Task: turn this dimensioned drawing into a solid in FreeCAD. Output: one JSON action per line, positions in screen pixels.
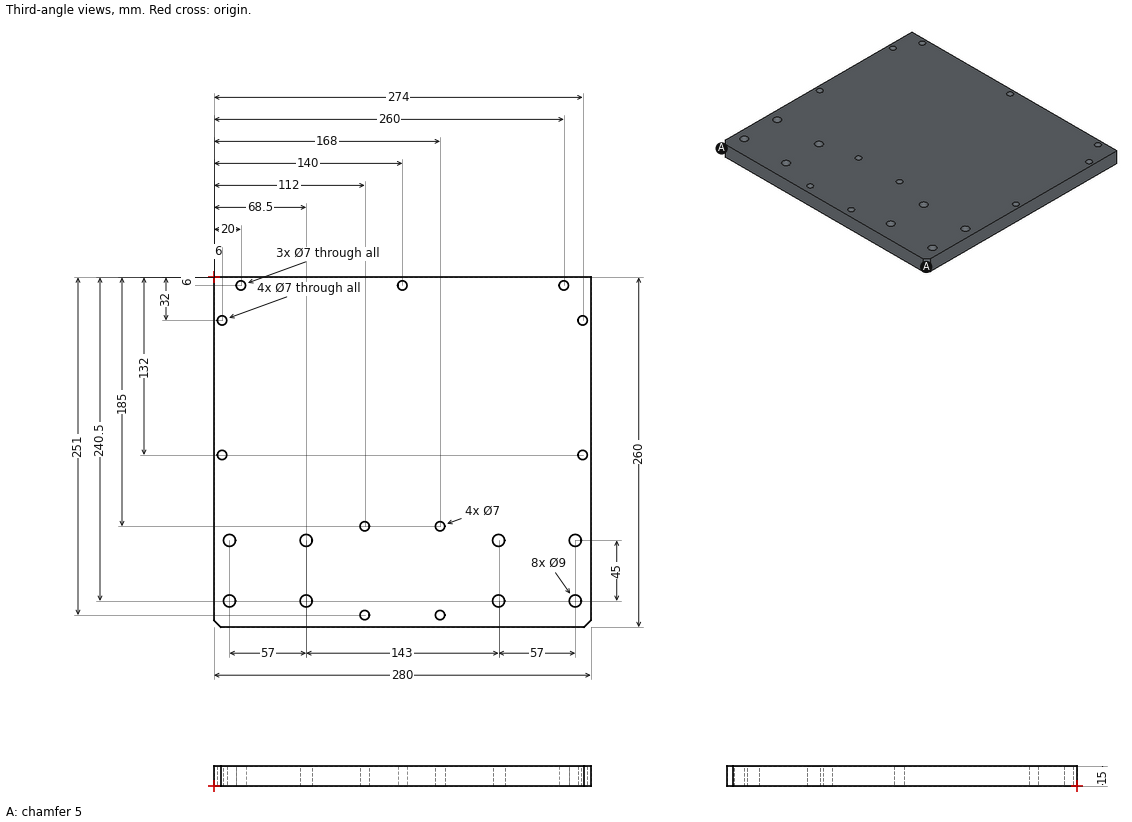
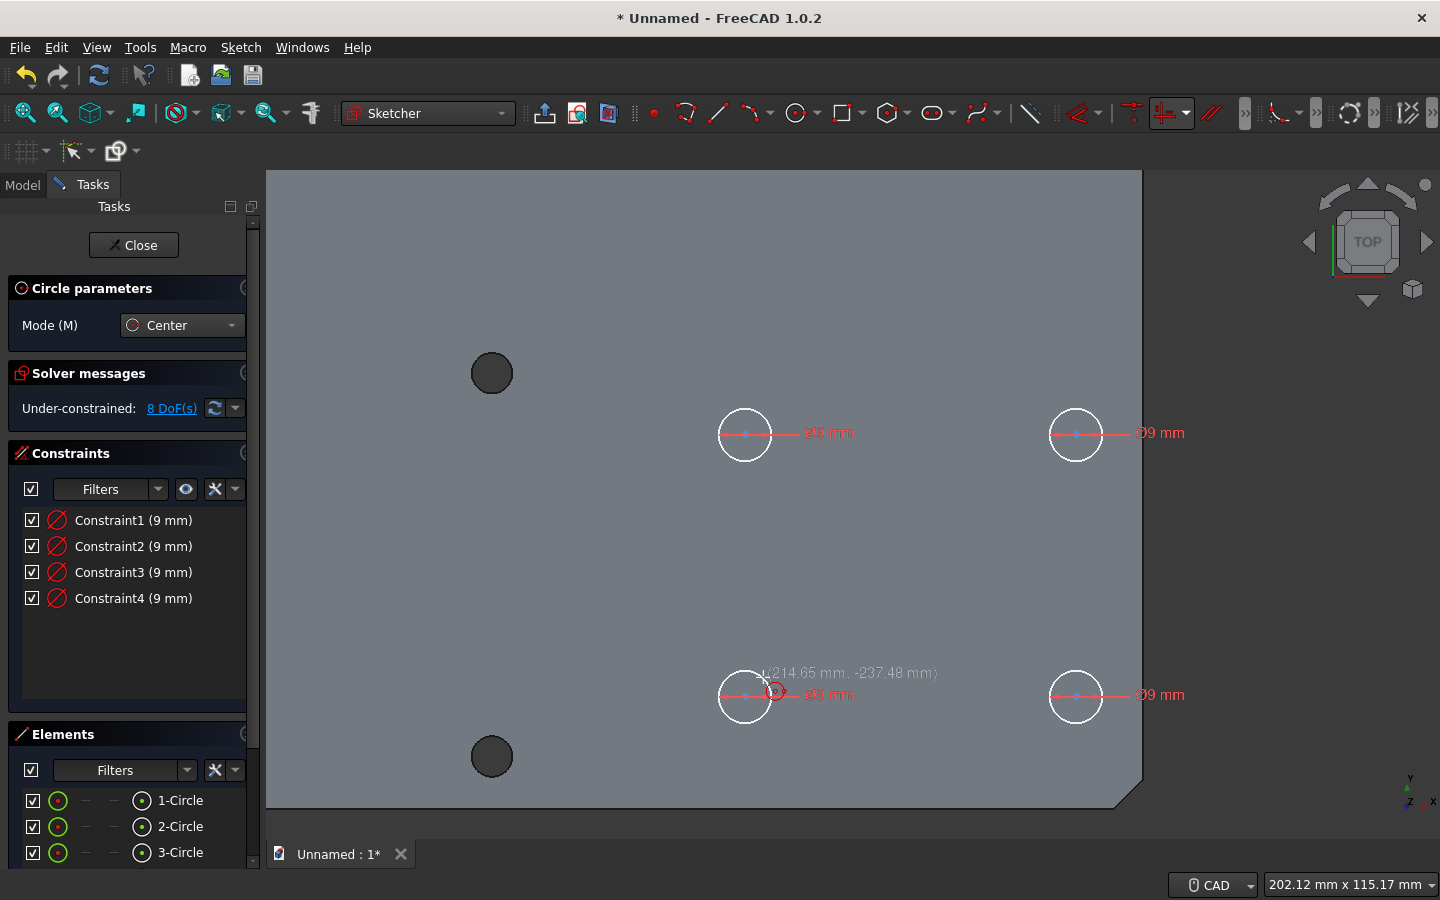
{"action": "scroll", "coordinate": [989, 718], "scroll_direction": "down", "scroll_amount": 6}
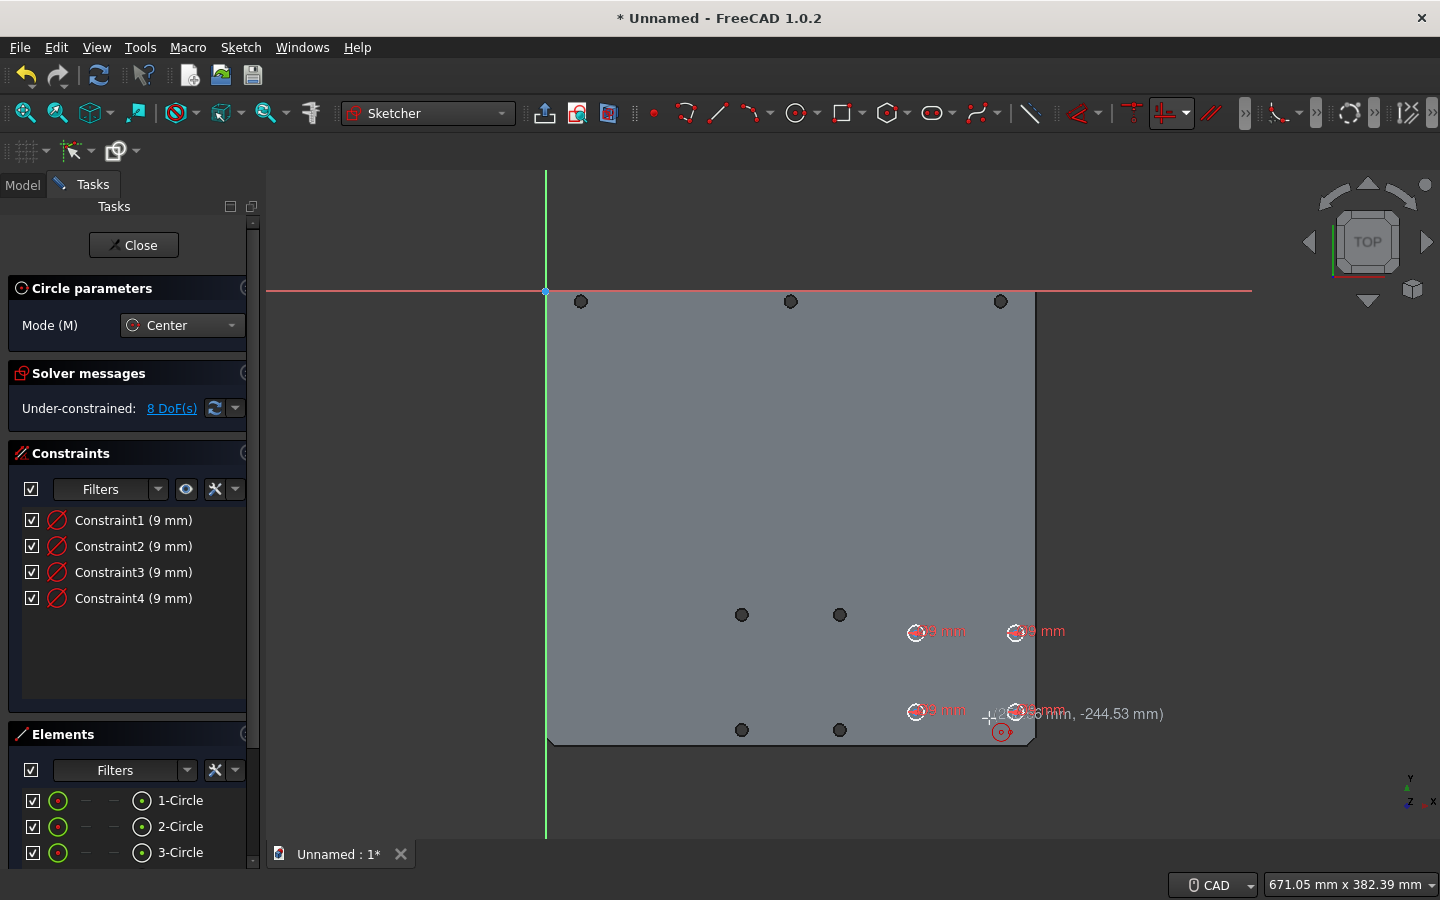
{"action": "scroll", "coordinate": [666, 712], "scroll_direction": "up", "scroll_amount": 6}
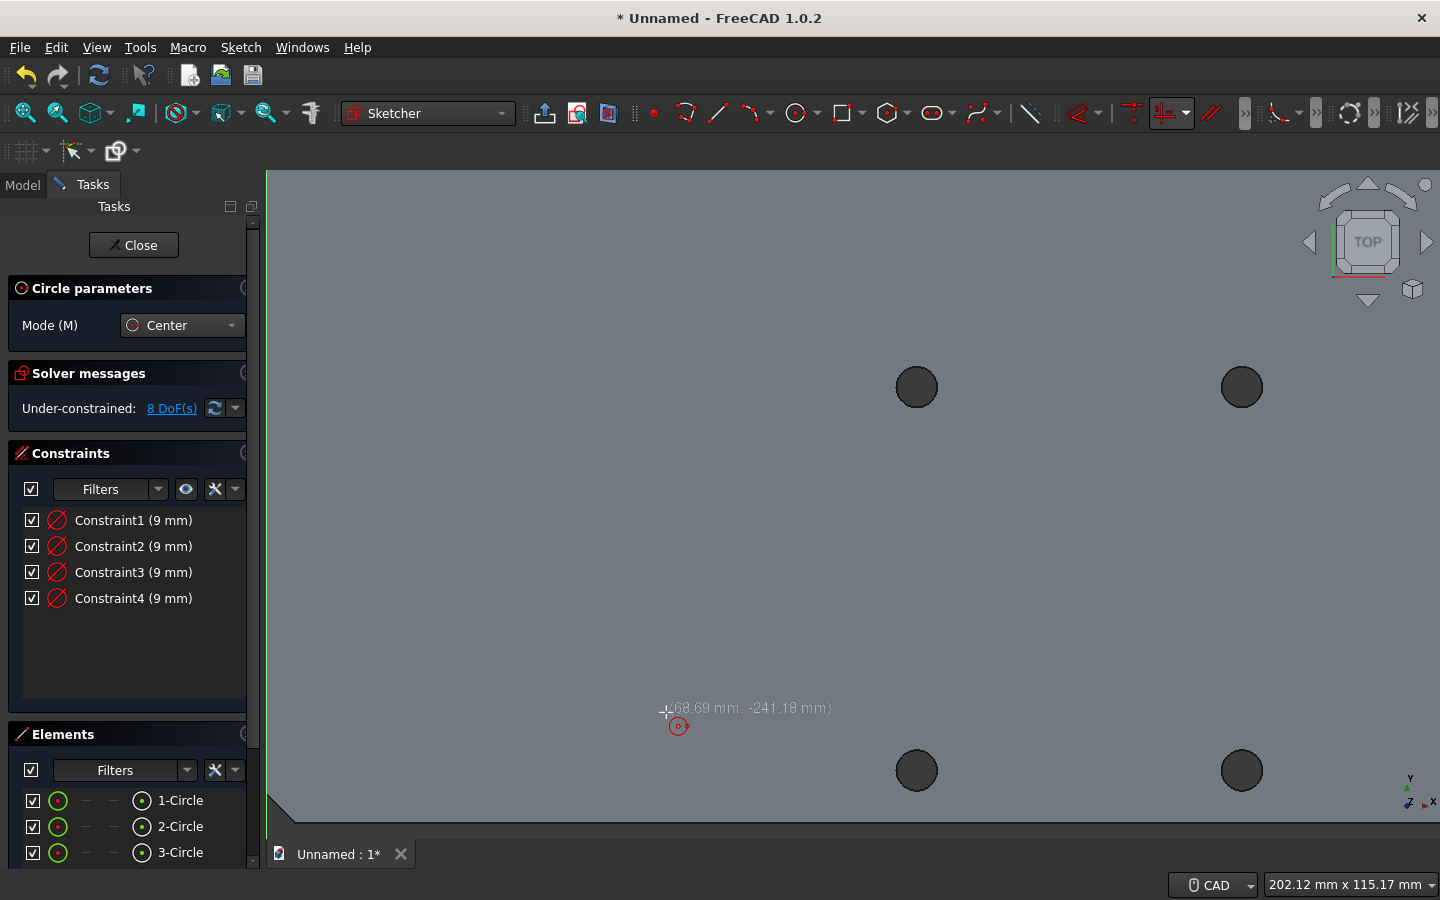
{"action": "left_click", "coordinate": [664, 710]}
{"action": "mouse_move", "coordinate": [683, 691]}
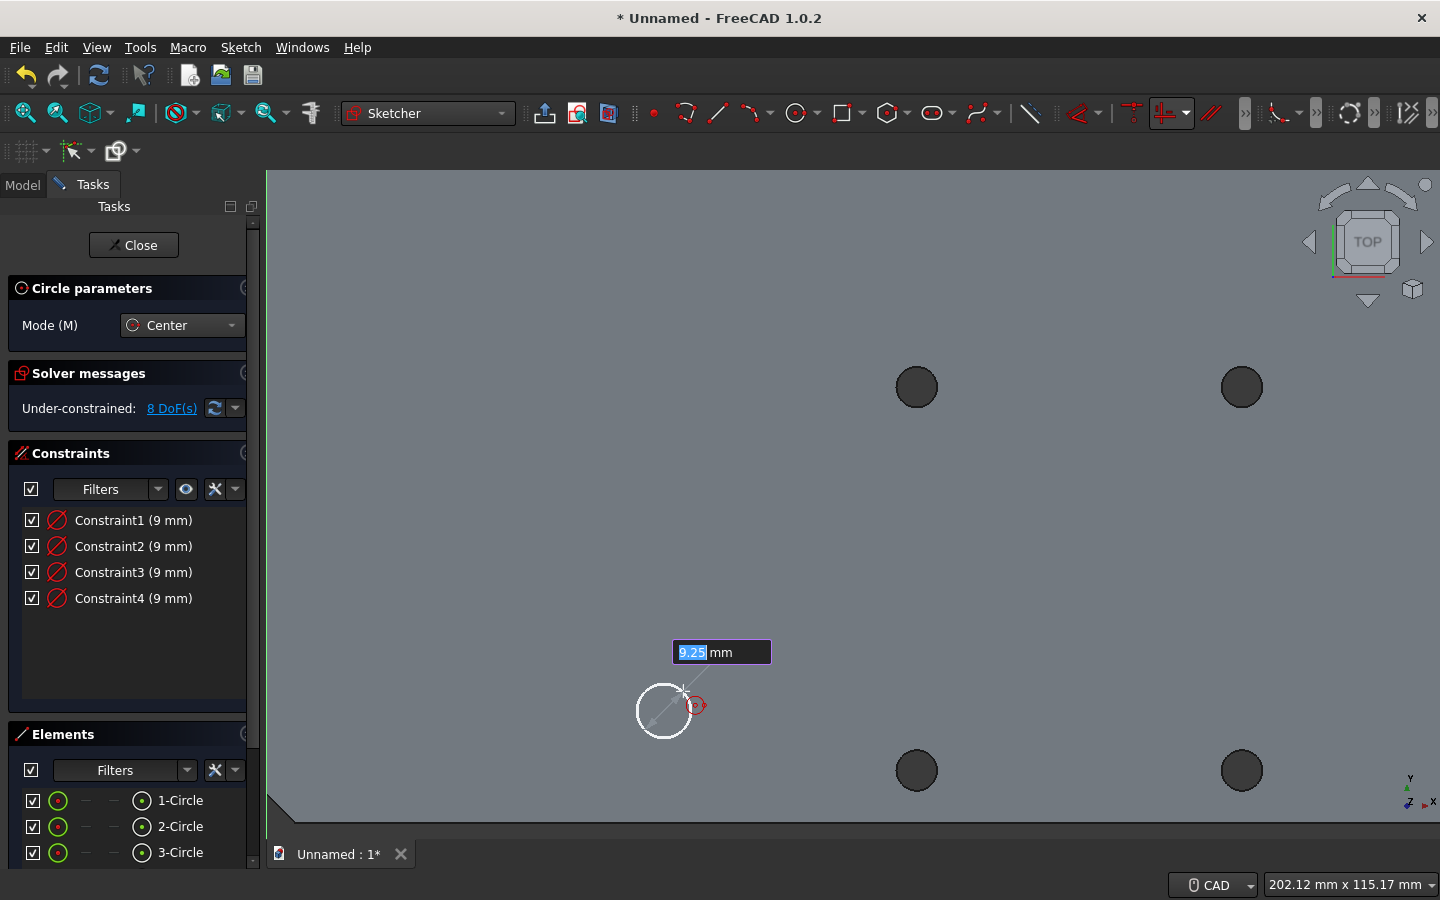
{"action": "type", "text": "9"}
{"action": "key", "text": "Return"}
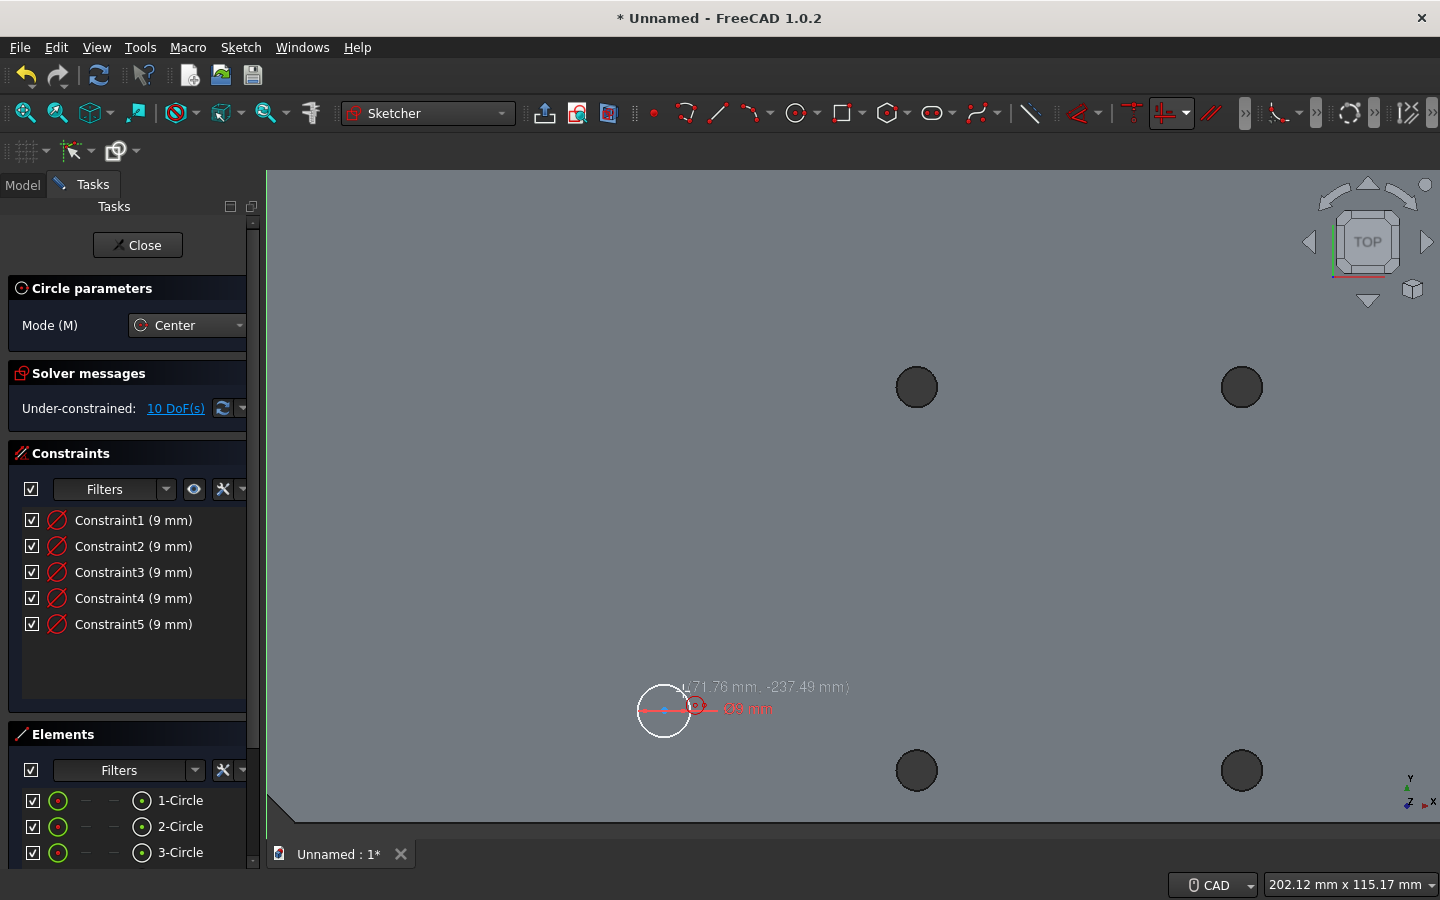
{"action": "left_click", "coordinate": [664, 448]}
{"action": "mouse_move", "coordinate": [683, 430]}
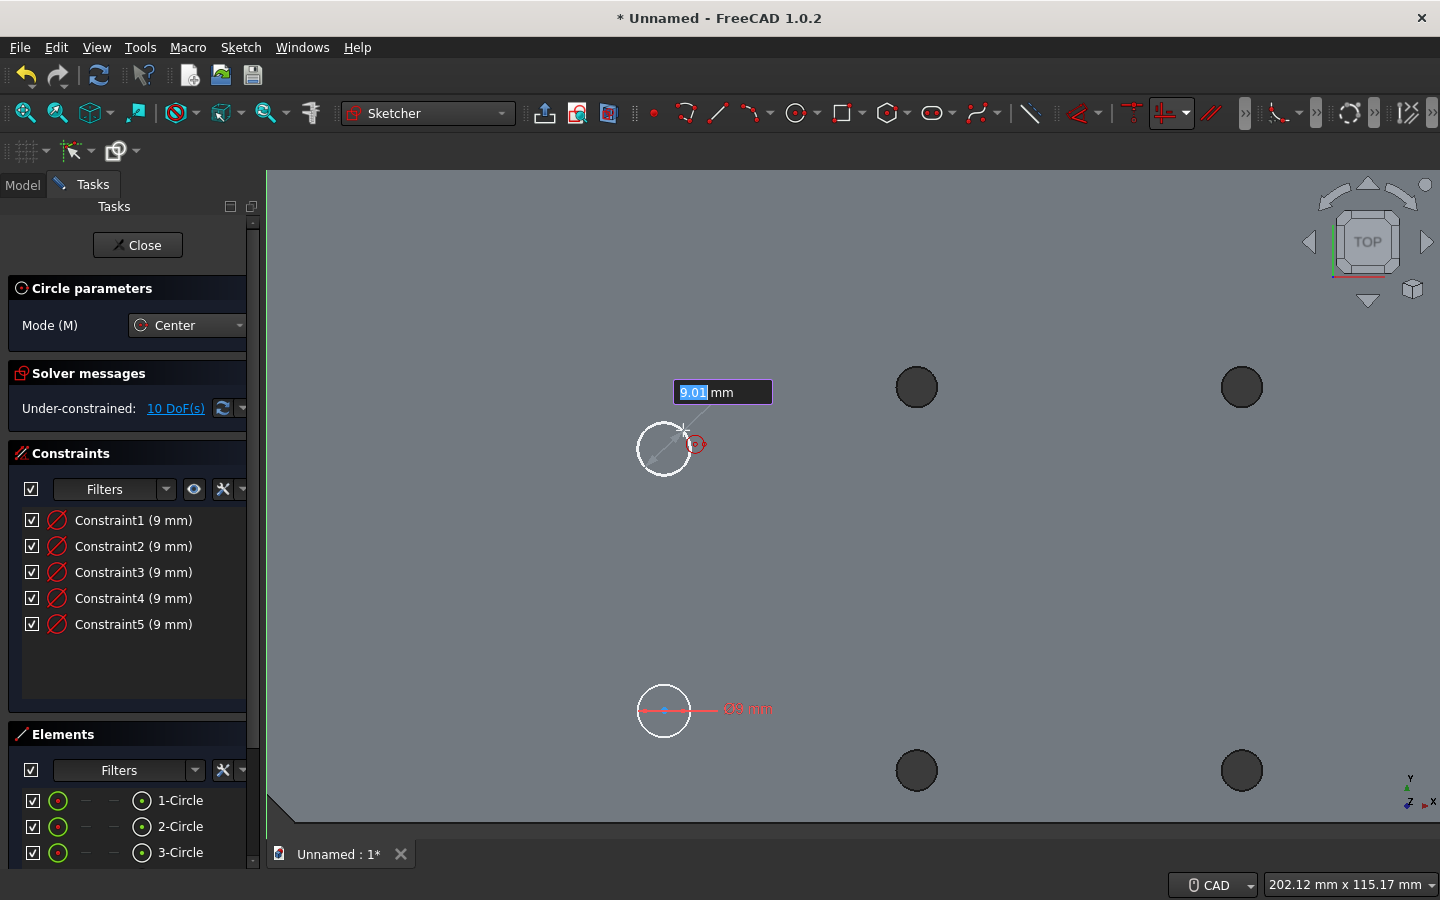
{"action": "type", "text": "9"}
{"action": "key", "text": "Return"}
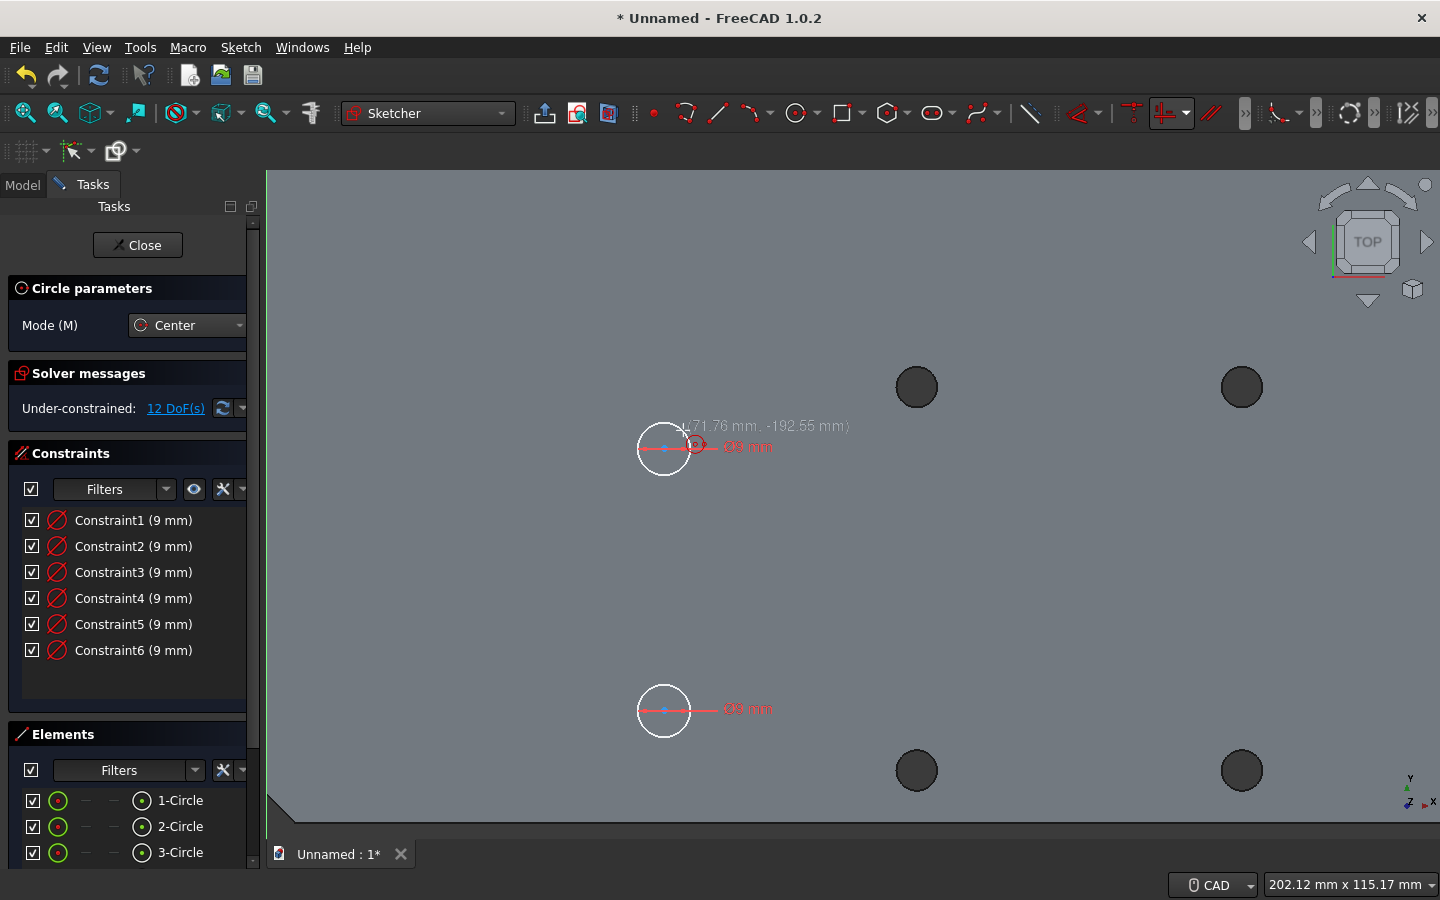
{"action": "left_click", "coordinate": [333, 448]}
{"action": "mouse_move", "coordinate": [351, 430]}